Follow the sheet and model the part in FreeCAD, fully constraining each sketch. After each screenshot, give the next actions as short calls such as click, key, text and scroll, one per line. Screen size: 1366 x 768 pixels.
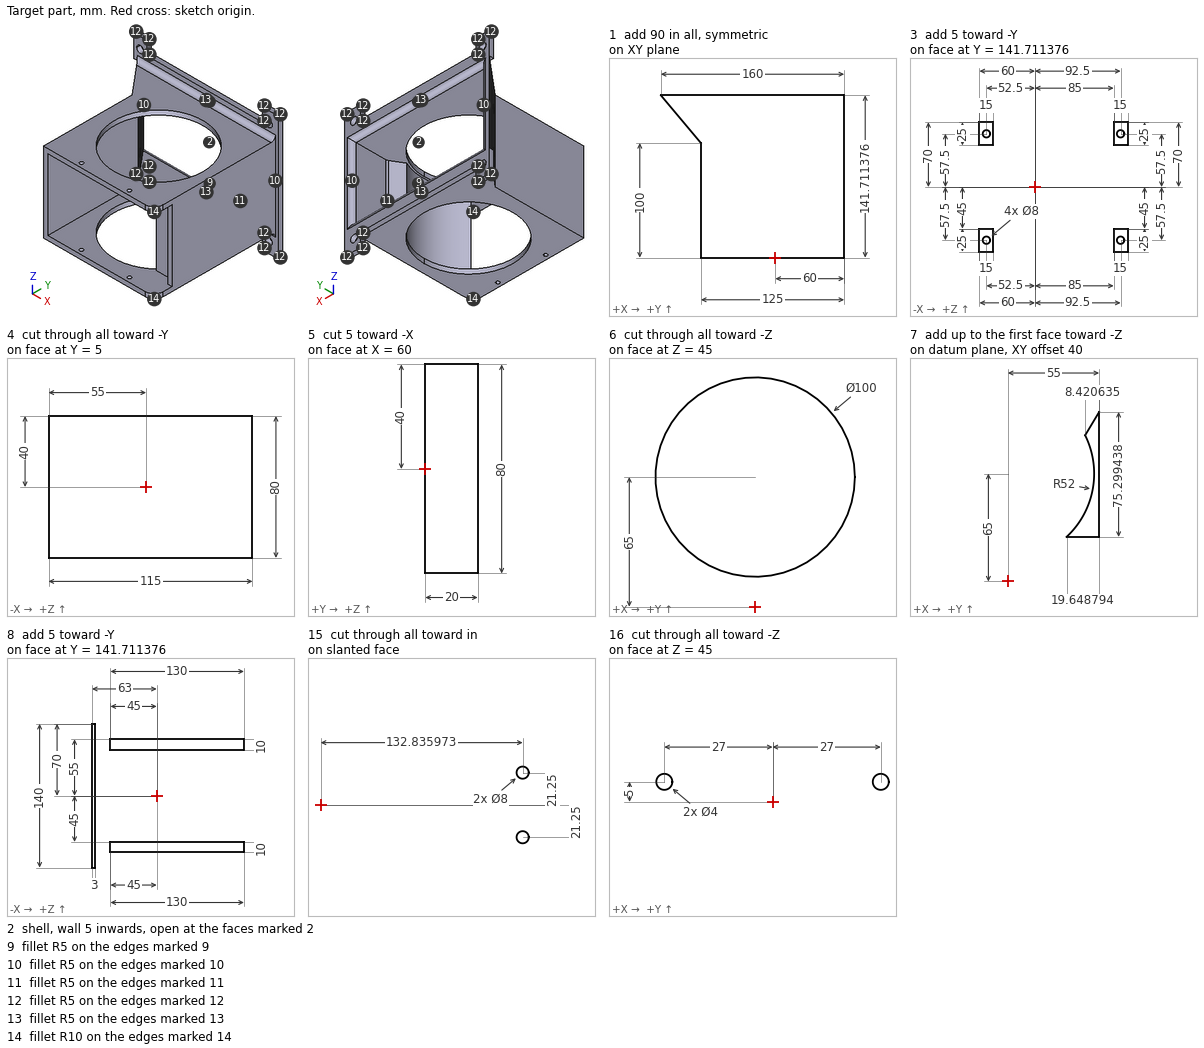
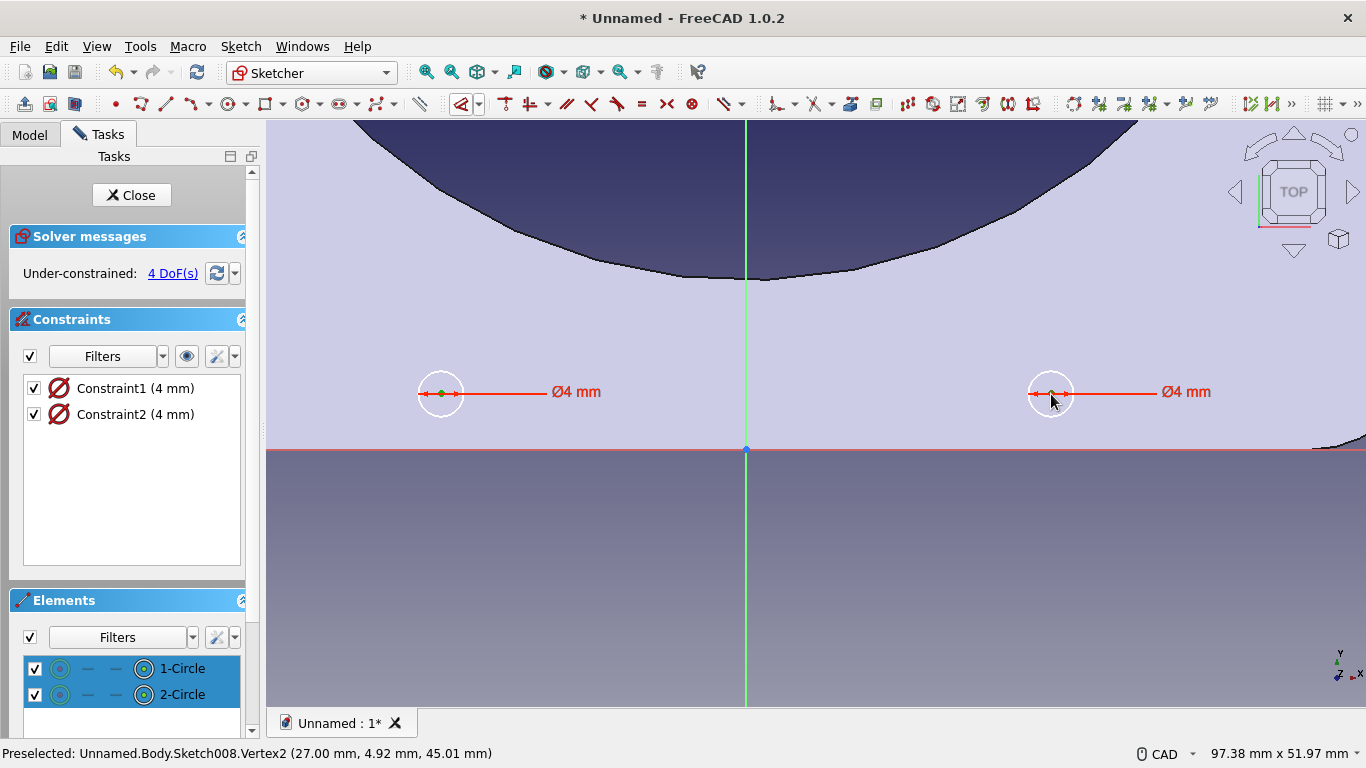
key(h)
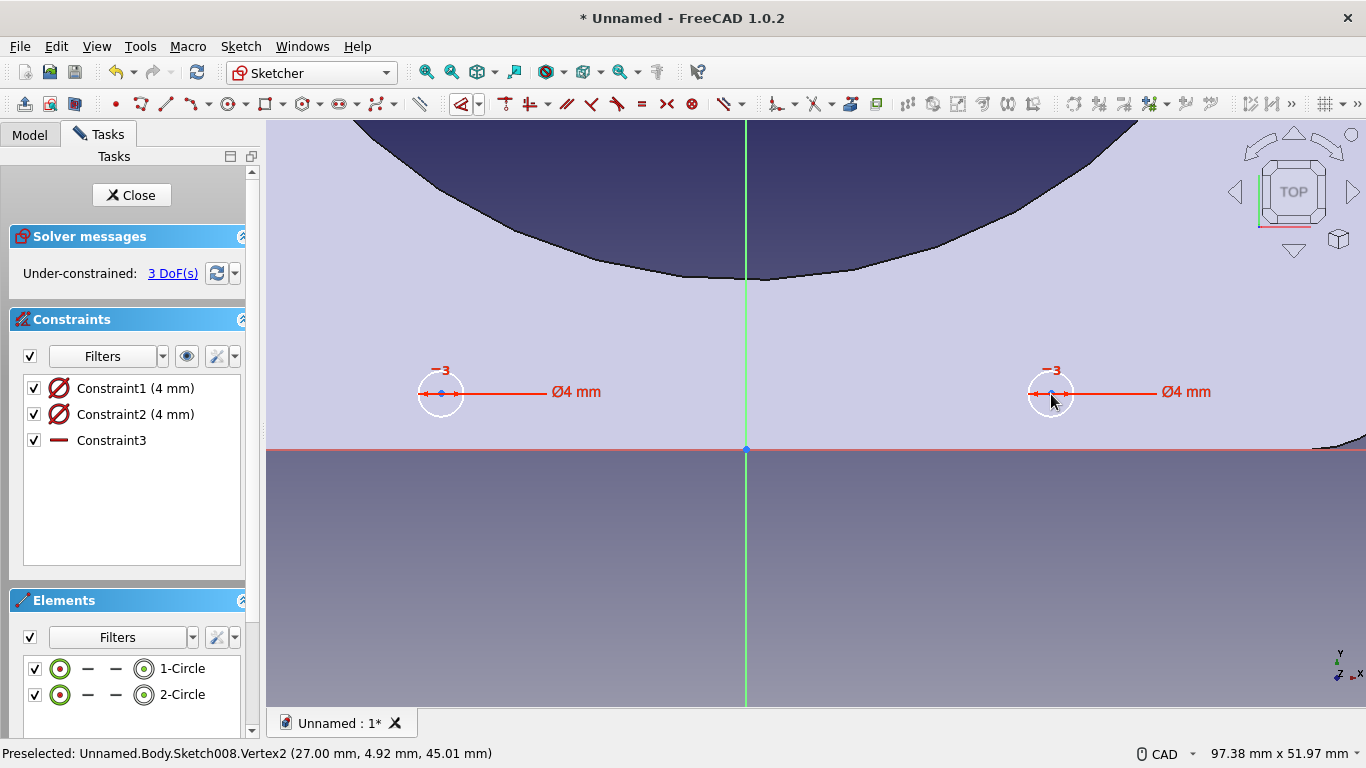
click(441, 394)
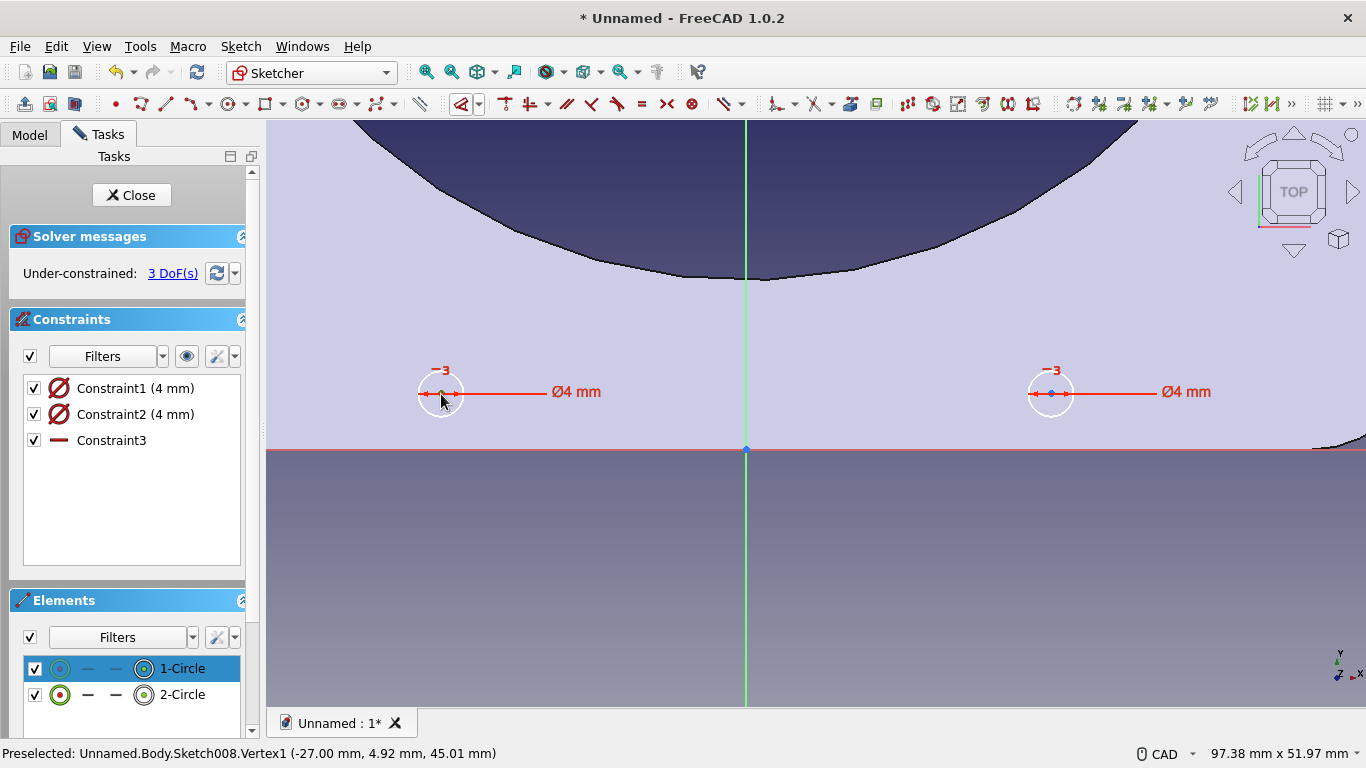
key(i)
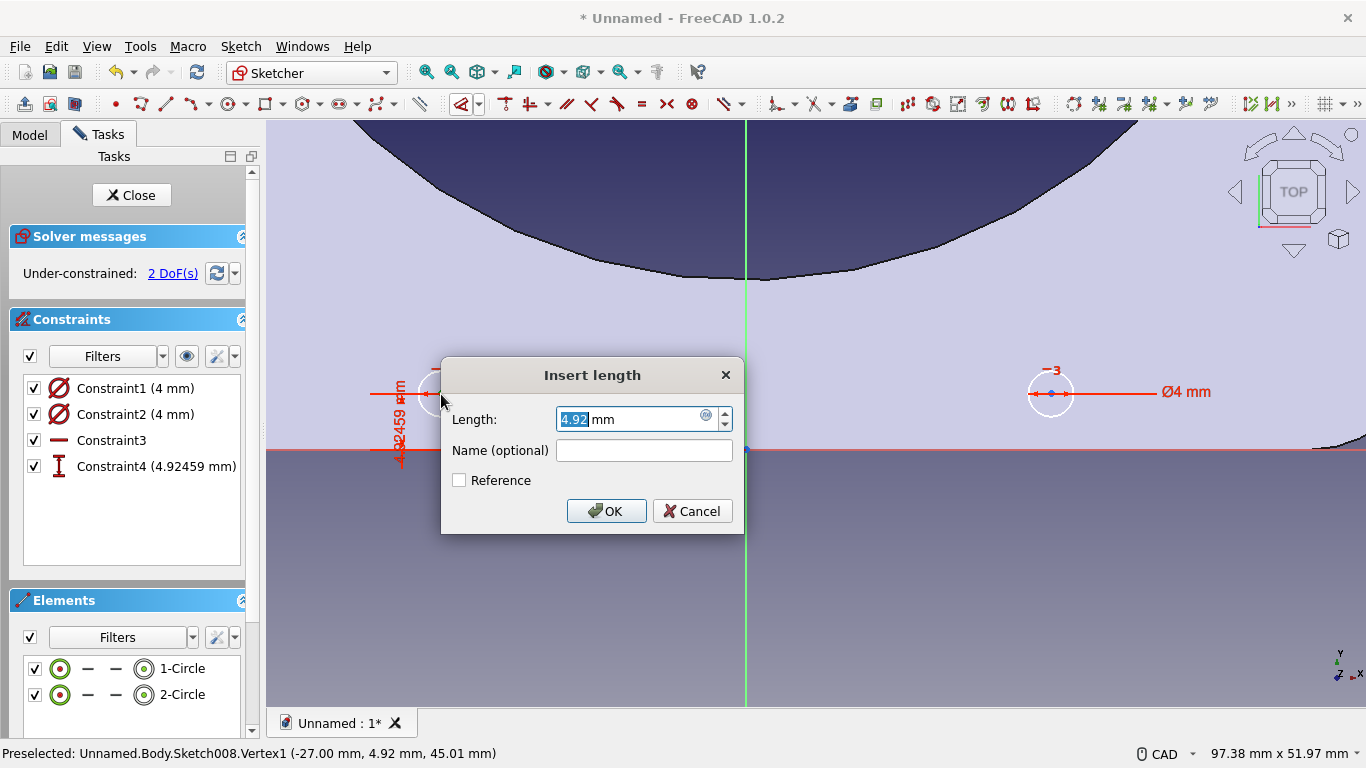
text(5)
key(Return)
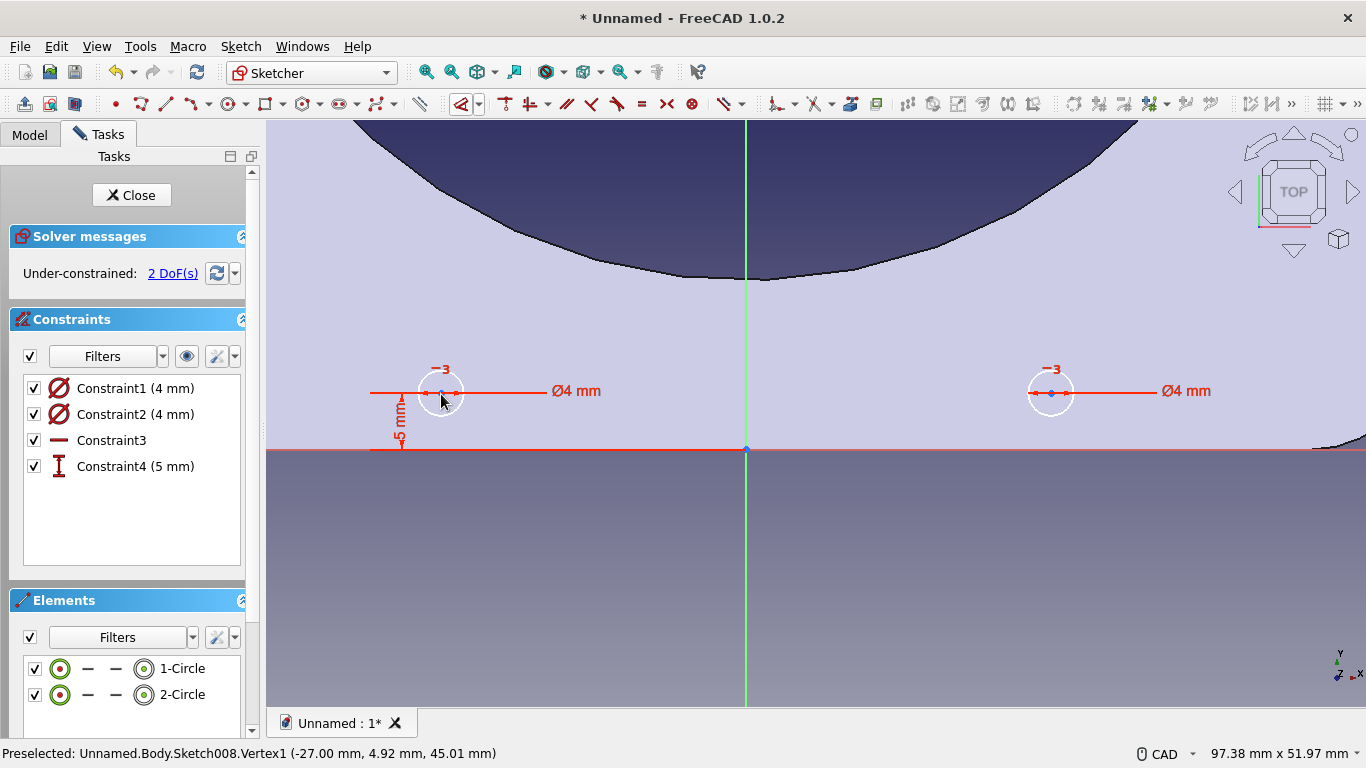
click(441, 393)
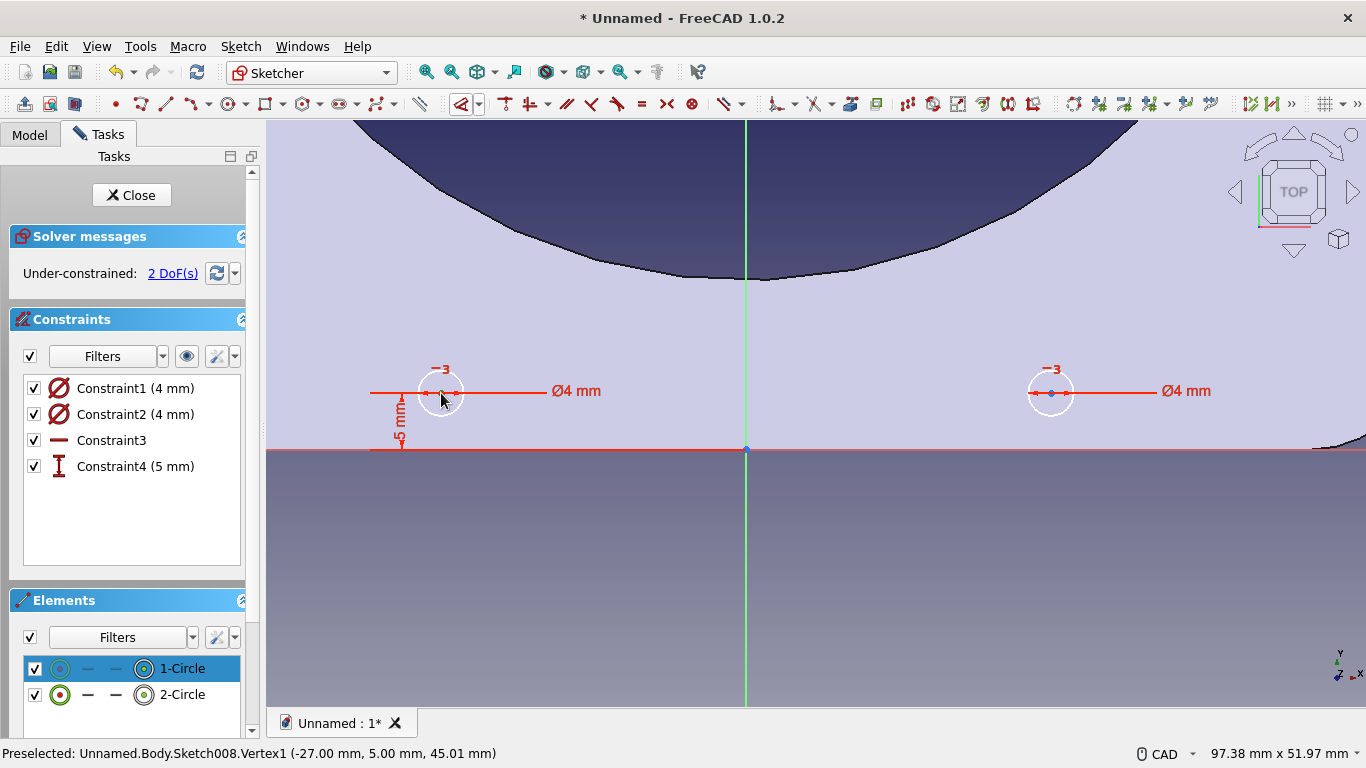
key(l)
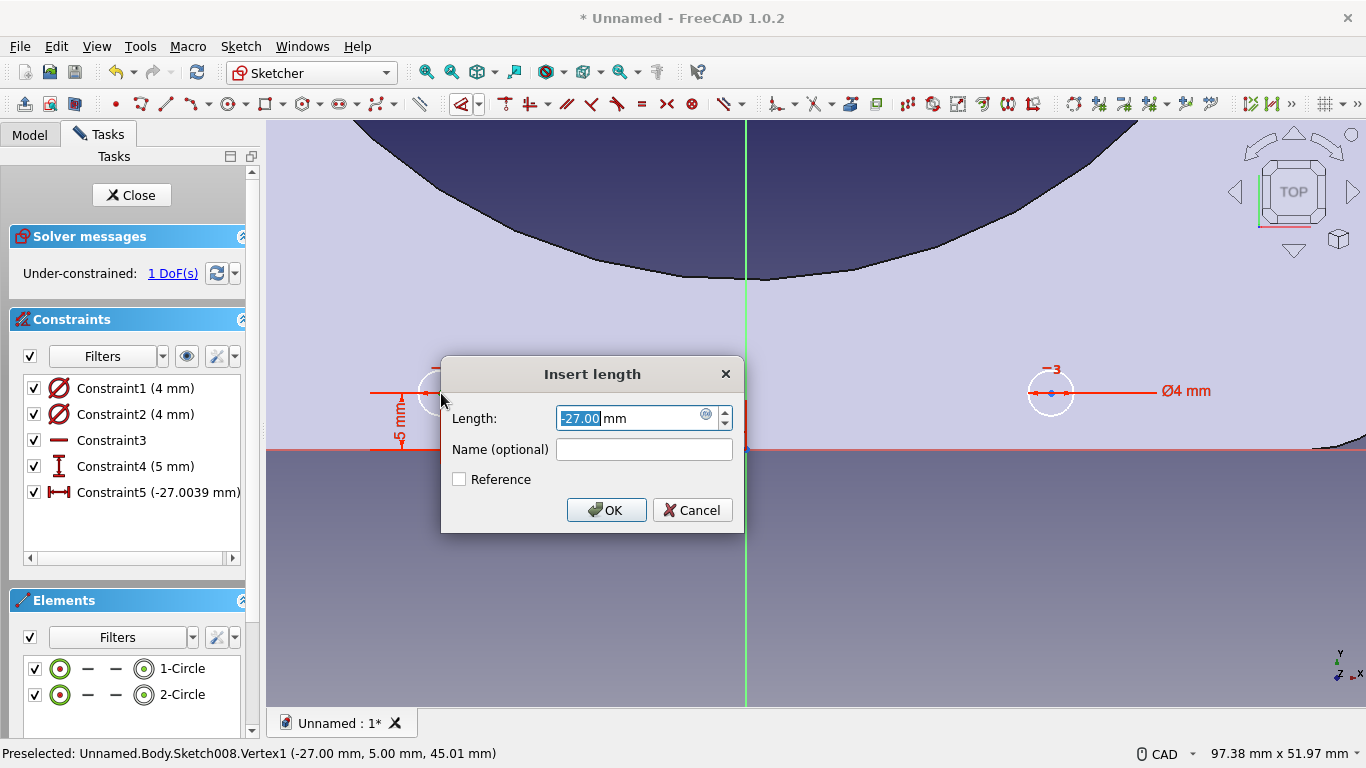
text(-27)
key(Return)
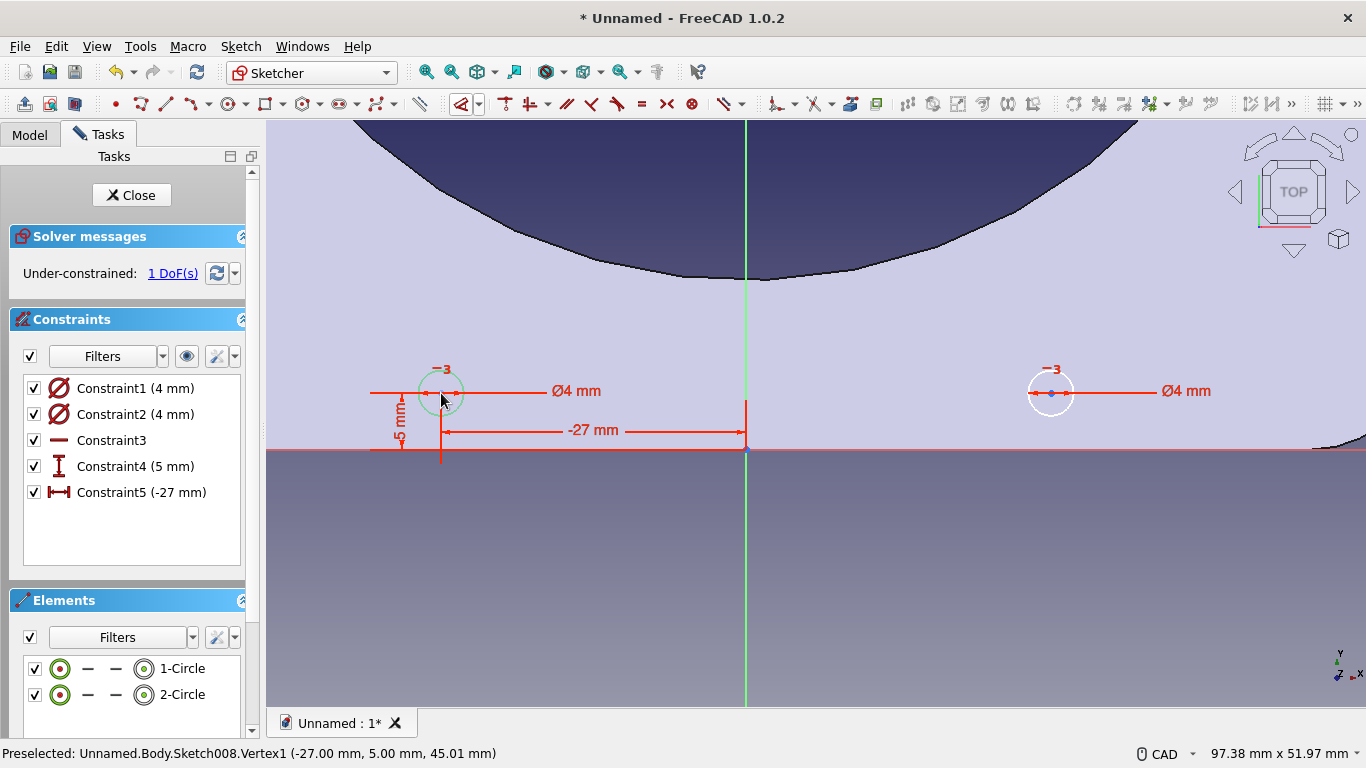
click(1051, 393)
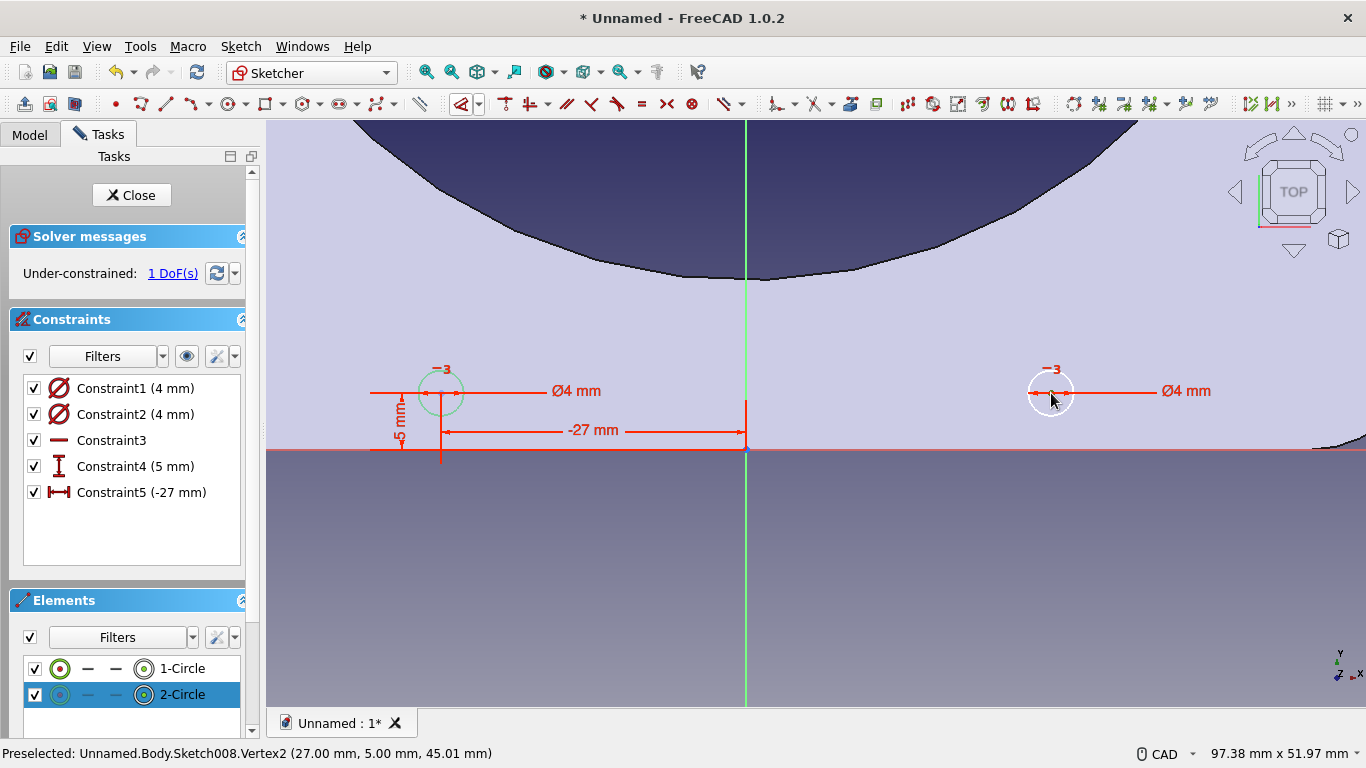
key(l)